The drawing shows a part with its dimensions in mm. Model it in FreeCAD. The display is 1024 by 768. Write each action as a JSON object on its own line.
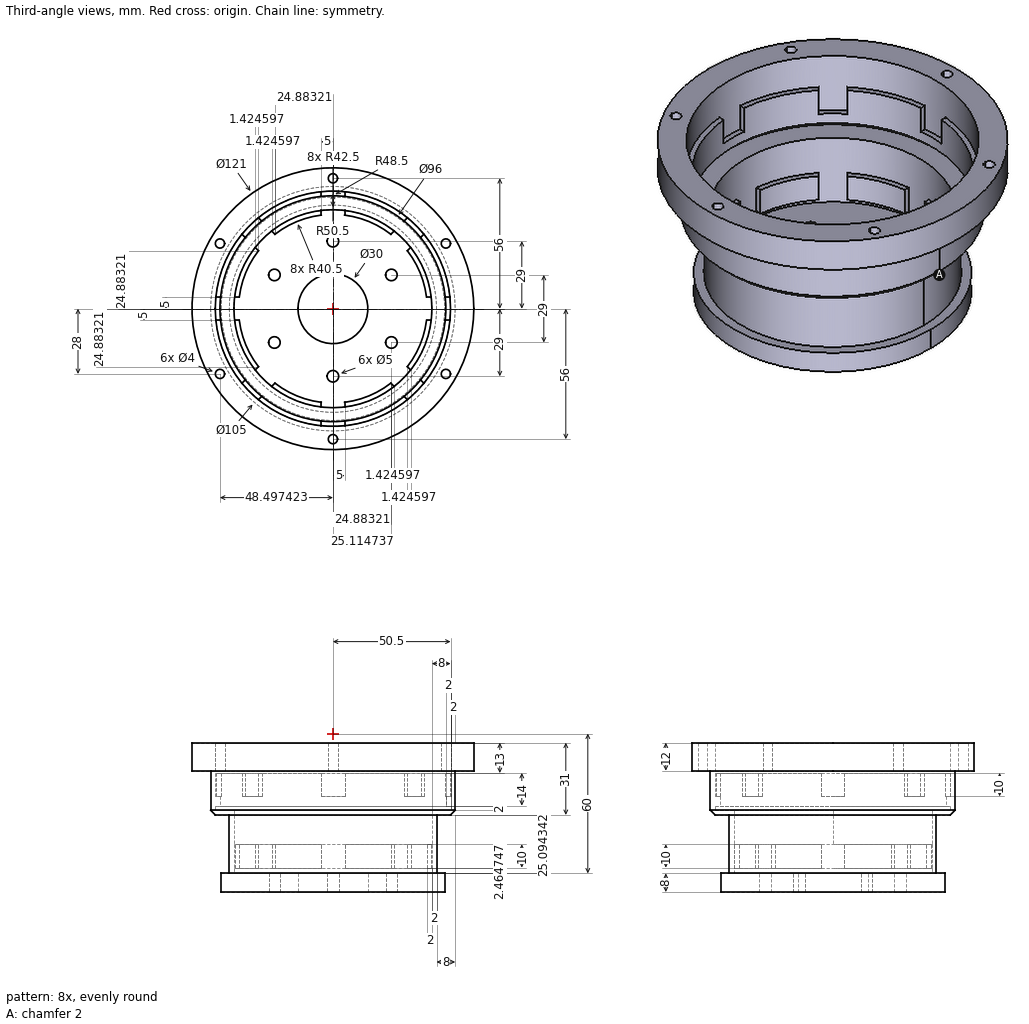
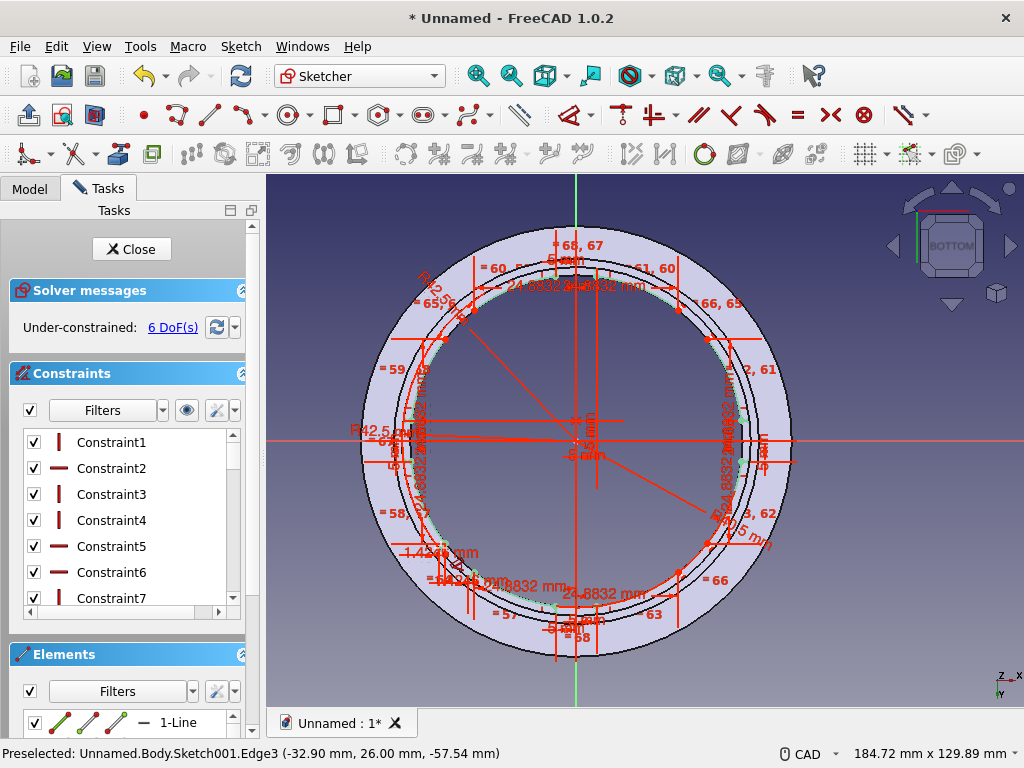
{"action": "scroll", "coordinate": [443, 338], "scroll_direction": "up", "scroll_amount": 10}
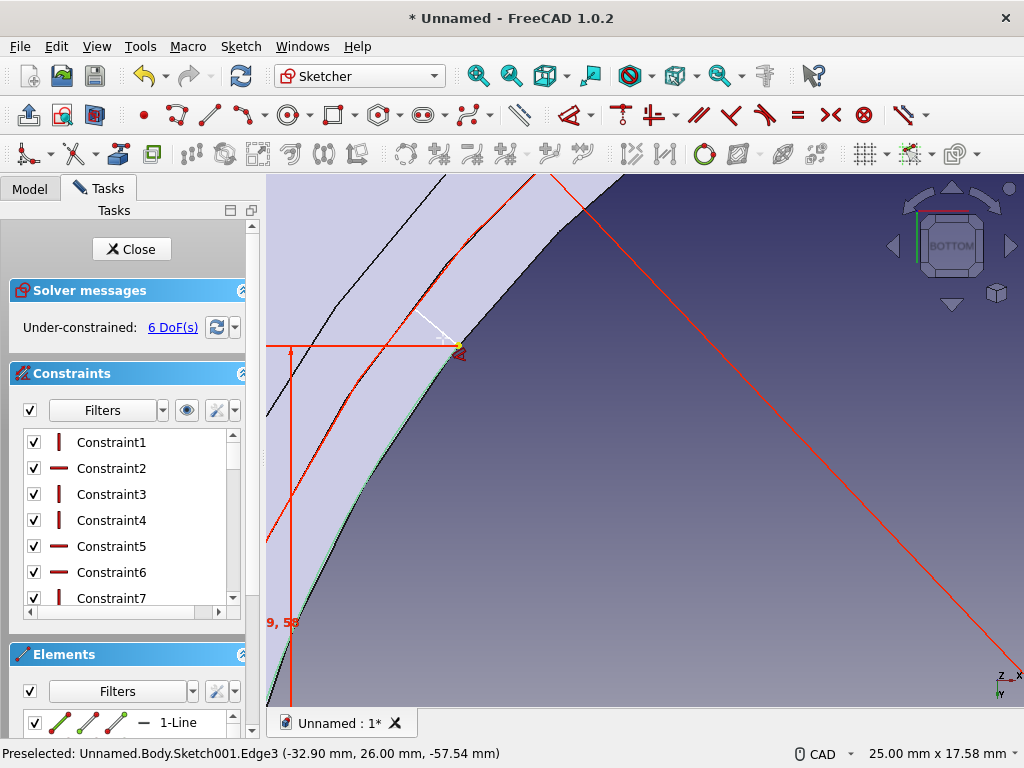
{"action": "left_click", "coordinate": [444, 334]}
{"action": "left_click", "coordinate": [419, 273]}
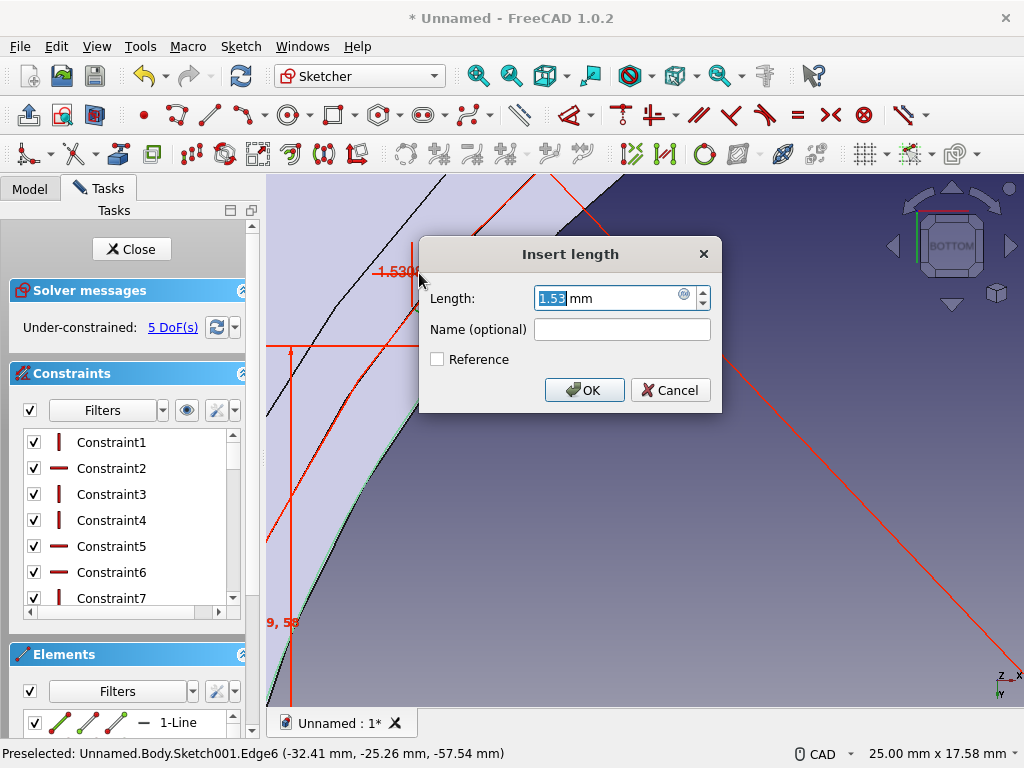
{"action": "type", "text": "1.424597"}
{"action": "key", "text": "Return"}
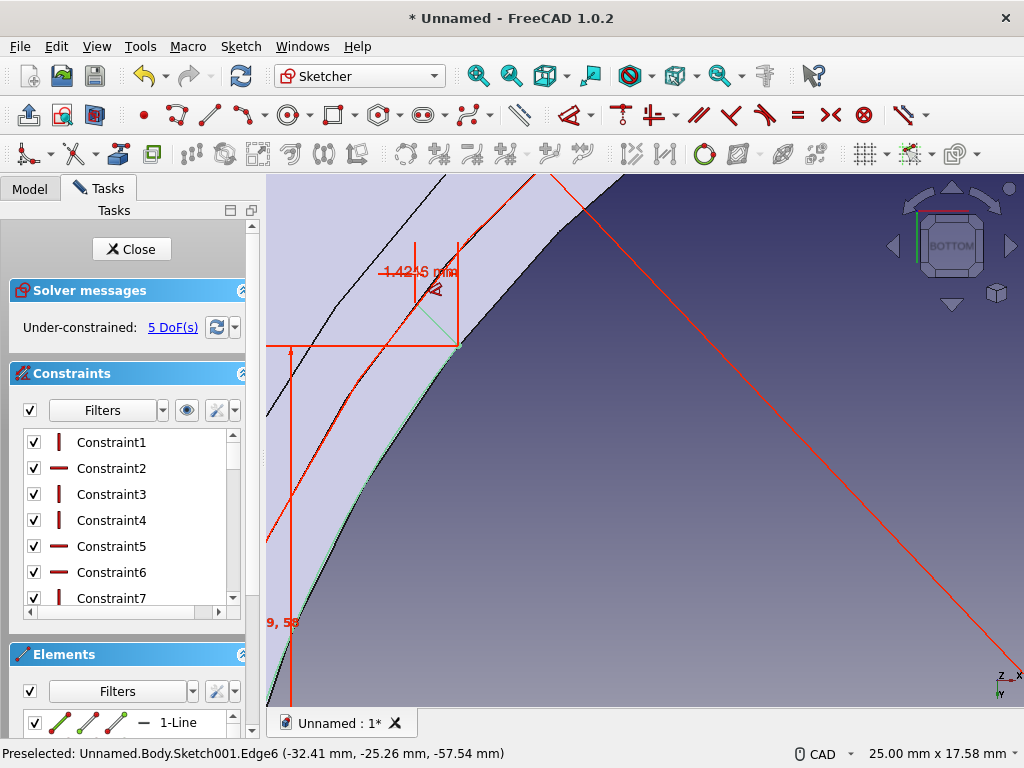
{"action": "scroll", "coordinate": [443, 337], "scroll_direction": "down", "scroll_amount": 10}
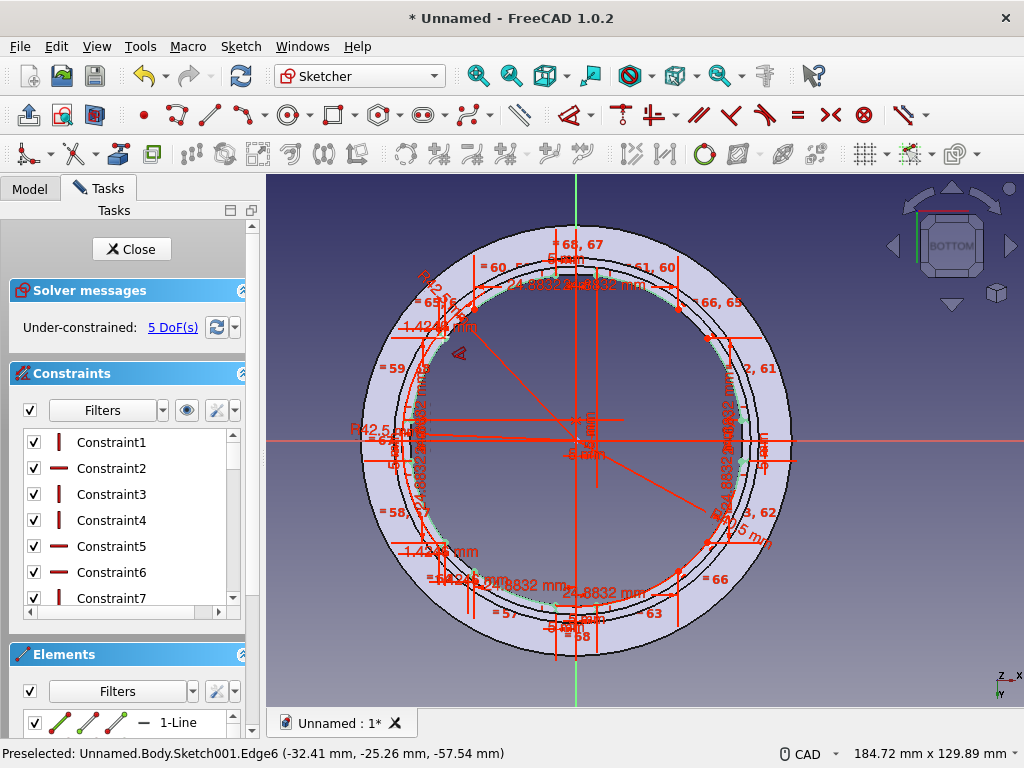
{"action": "scroll", "coordinate": [470, 305], "scroll_direction": "up", "scroll_amount": 10}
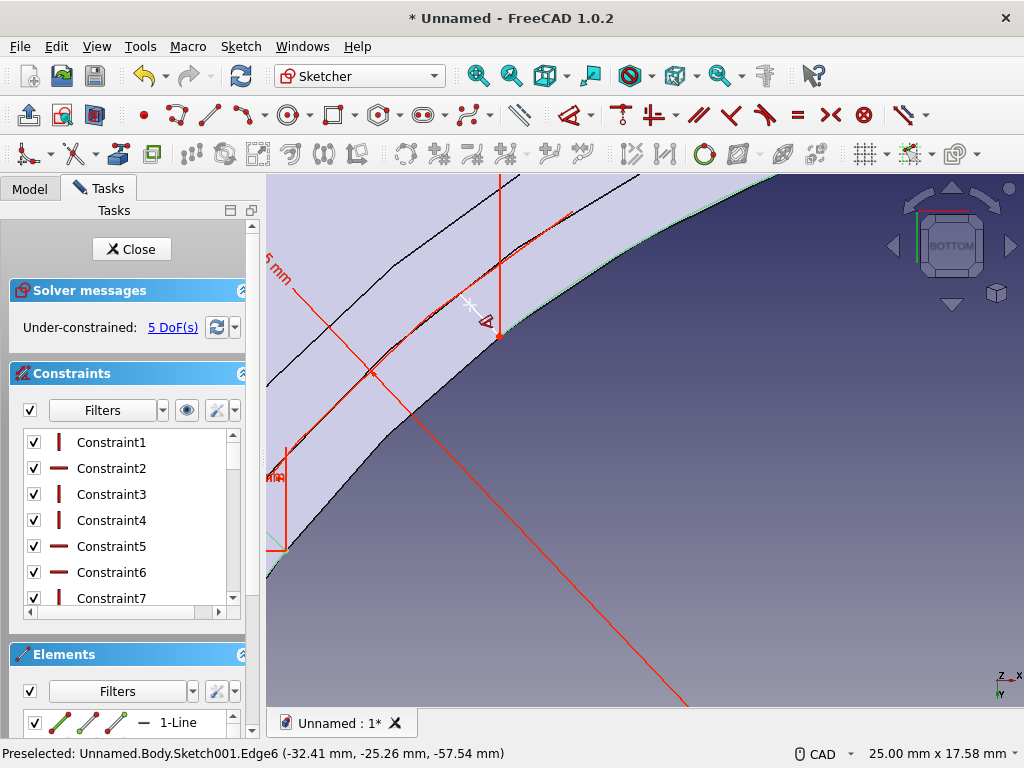
{"action": "left_click", "coordinate": [471, 305]}
{"action": "left_click", "coordinate": [479, 258]}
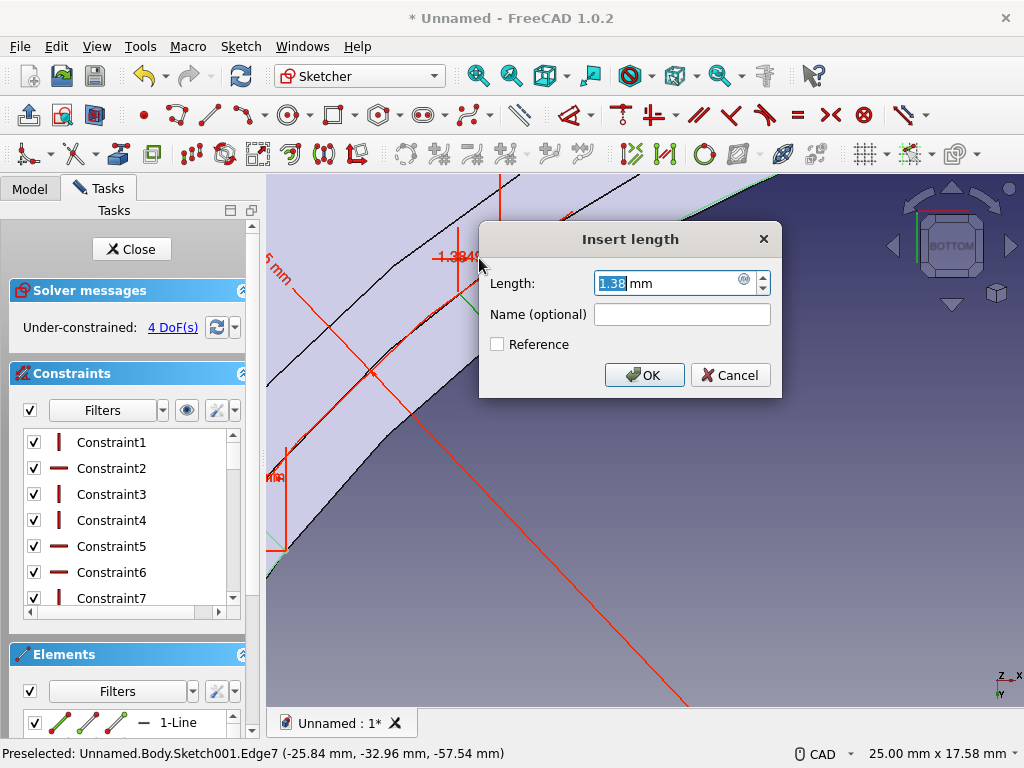
{"action": "type", "text": "1.424597"}
{"action": "key", "text": "Return"}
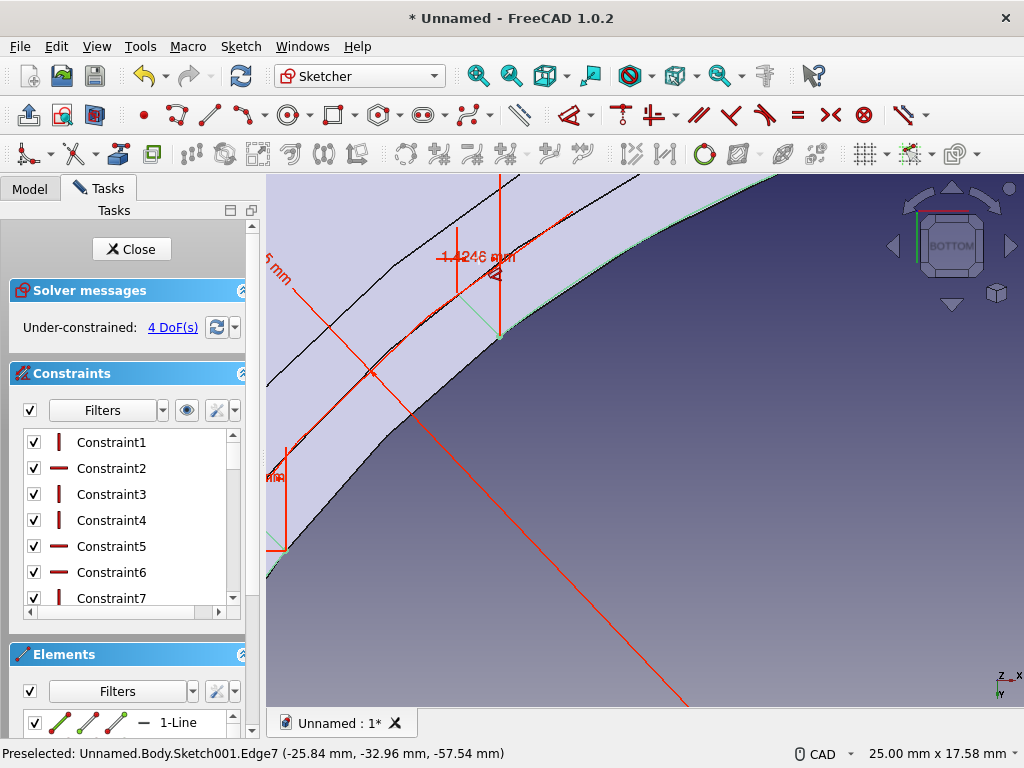
{"action": "scroll", "coordinate": [470, 305], "scroll_direction": "down", "scroll_amount": 10}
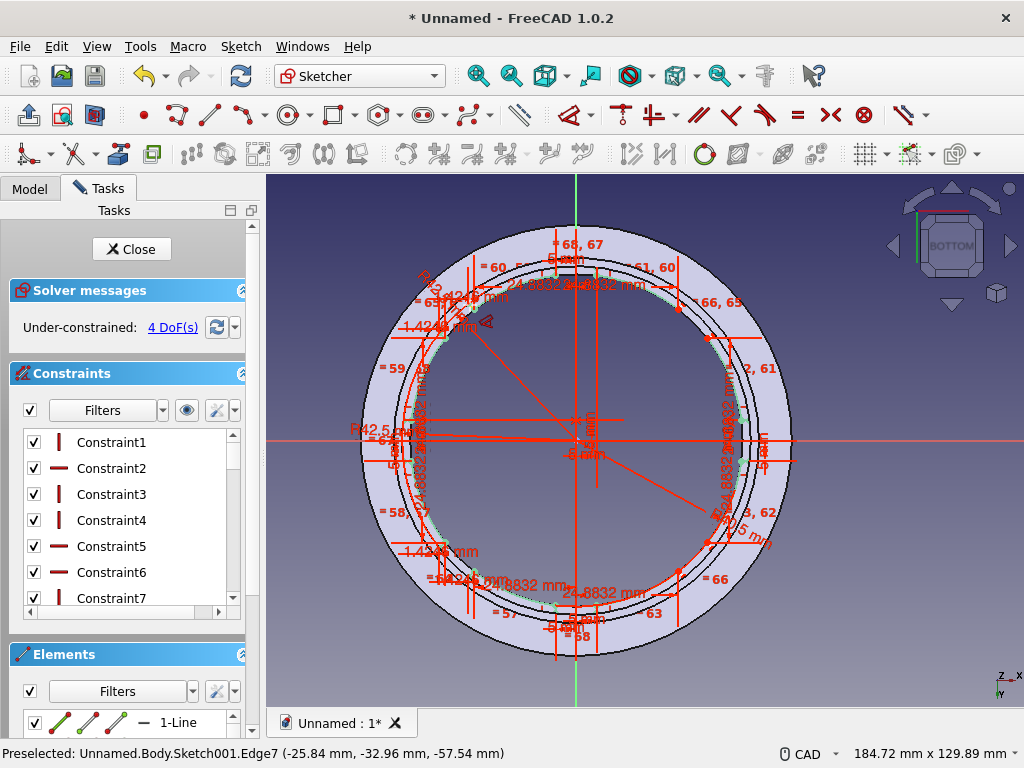
{"action": "scroll", "coordinate": [680, 308], "scroll_direction": "up", "scroll_amount": 10}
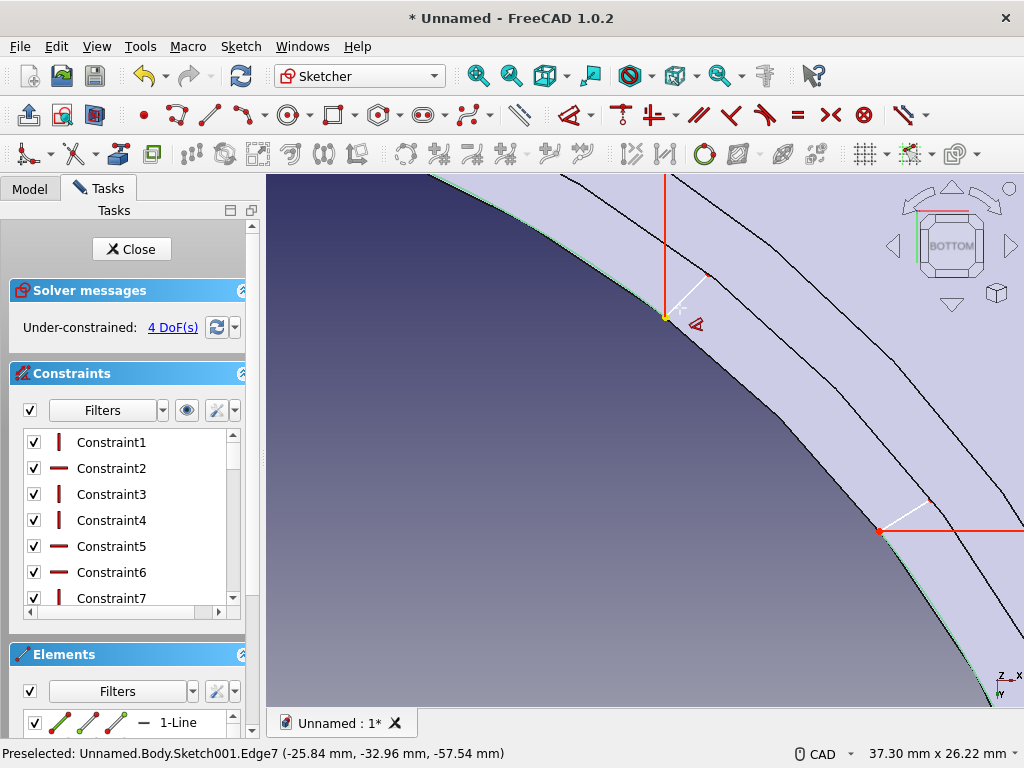
{"action": "left_click", "coordinate": [678, 304]}
{"action": "left_click", "coordinate": [687, 240]}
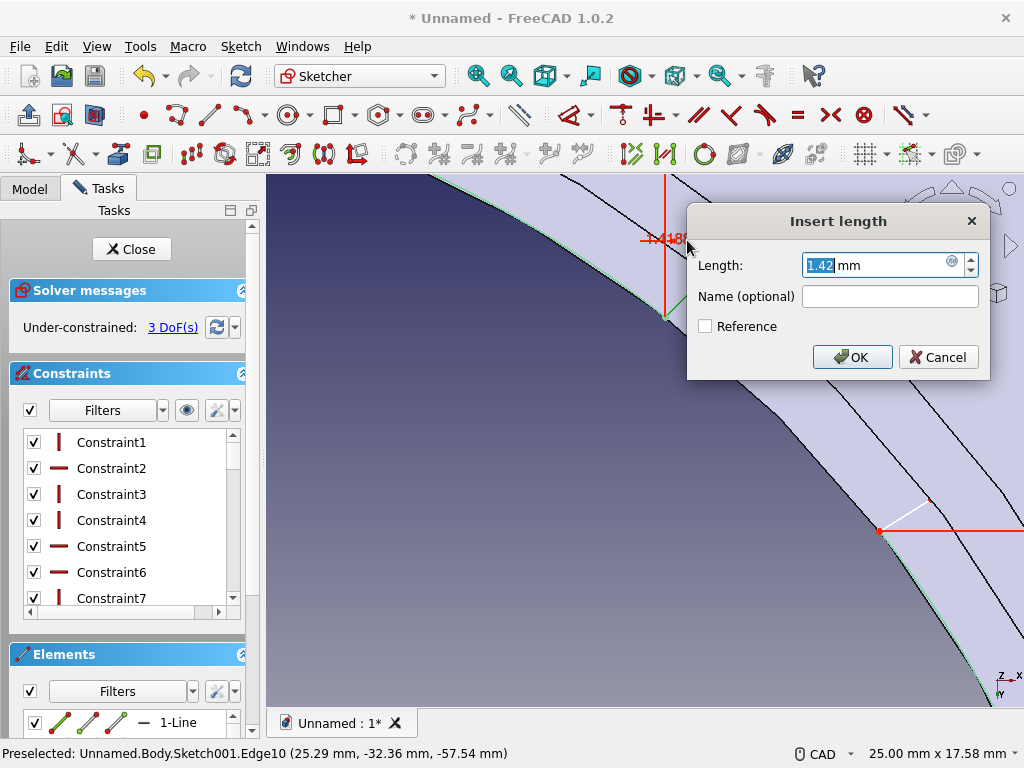
{"action": "type", "text": "1.424597"}
{"action": "key", "text": "Return"}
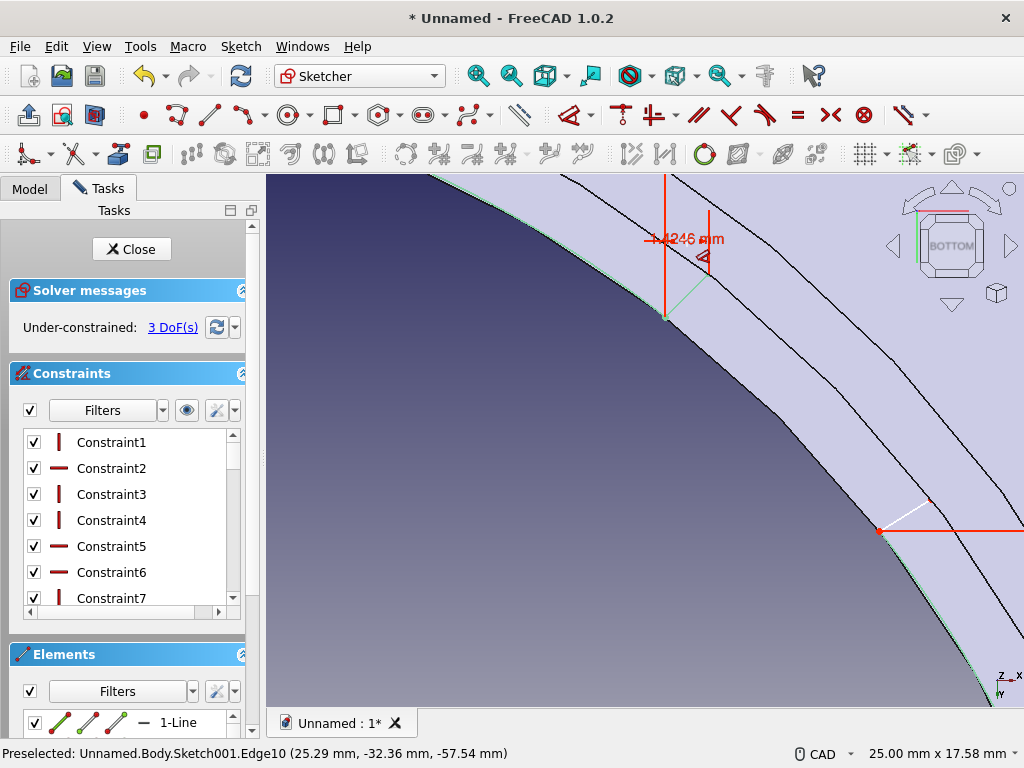
{"action": "scroll", "coordinate": [681, 308], "scroll_direction": "down", "scroll_amount": 10}